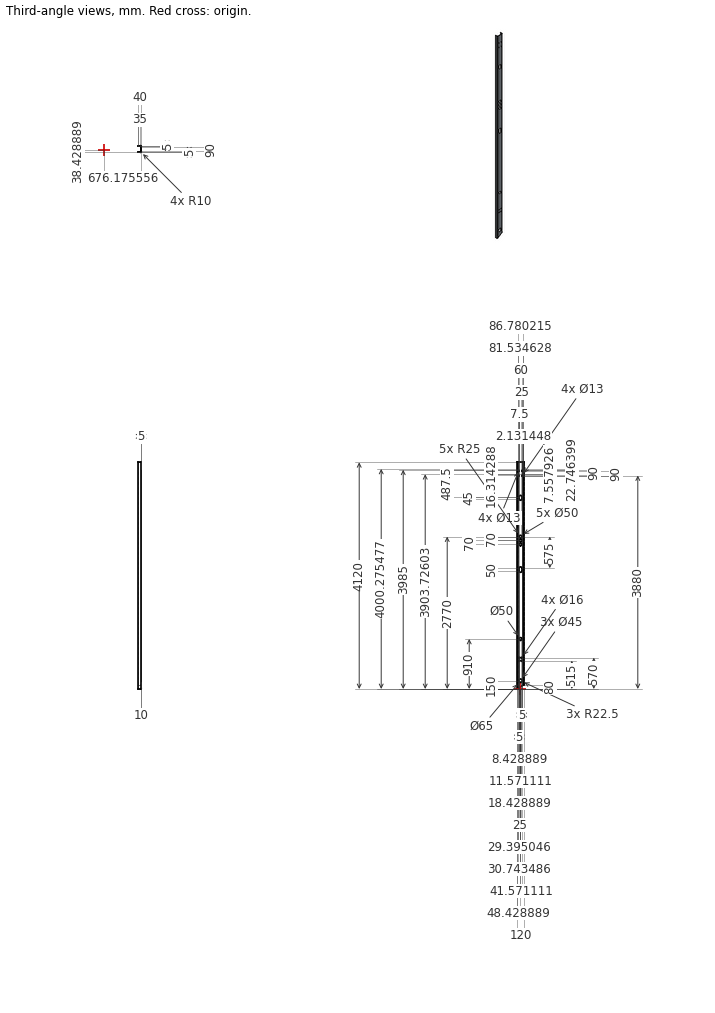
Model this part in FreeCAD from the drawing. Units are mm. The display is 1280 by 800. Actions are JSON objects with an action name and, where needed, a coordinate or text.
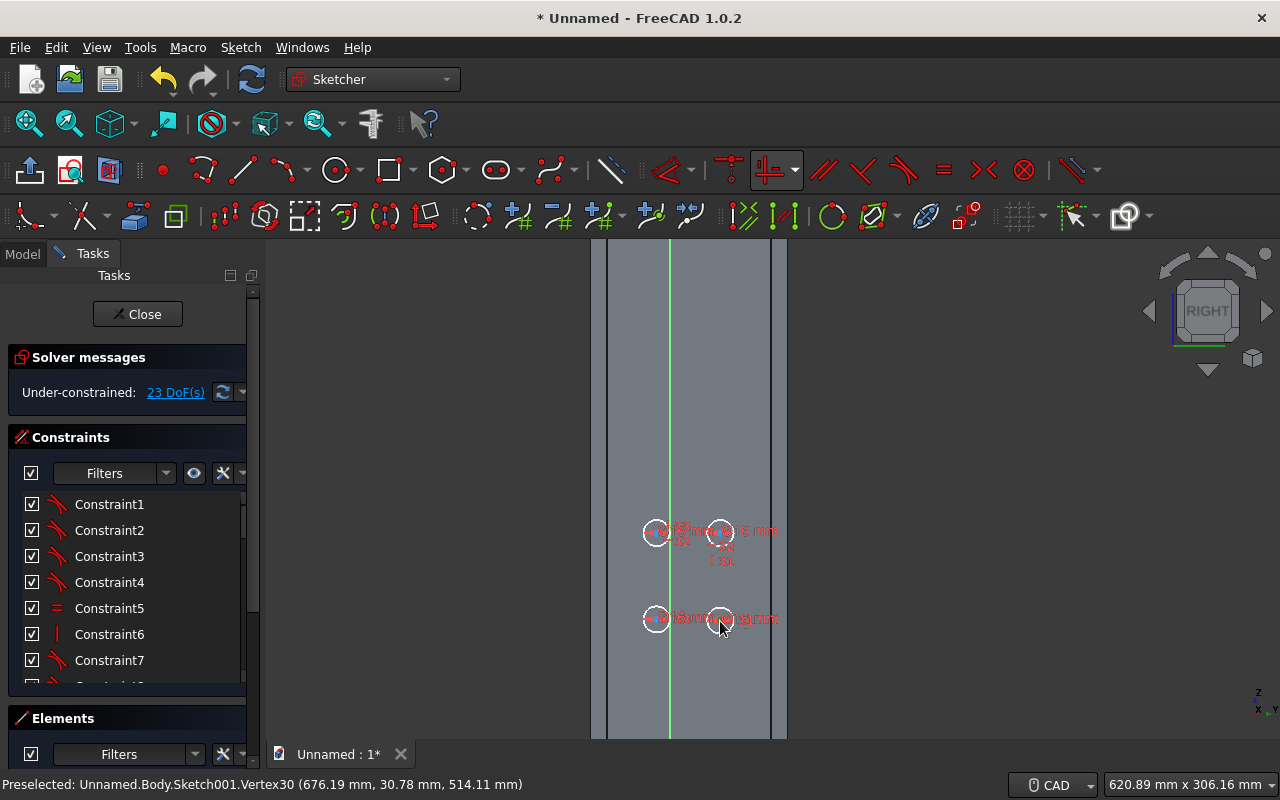
{"action": "scroll", "coordinate": [705, 609], "scroll_direction": "down", "scroll_amount": 15}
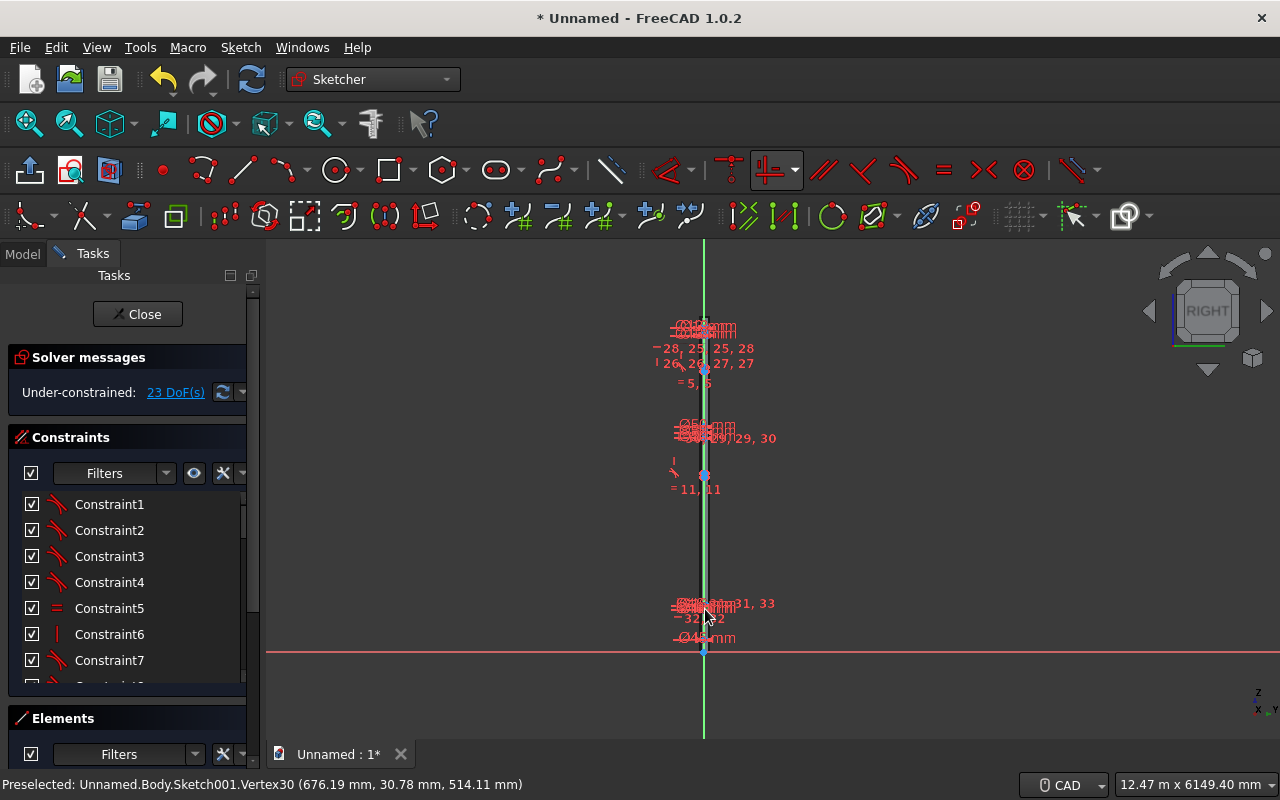
{"action": "scroll", "coordinate": [703, 610], "scroll_direction": "up", "scroll_amount": 7}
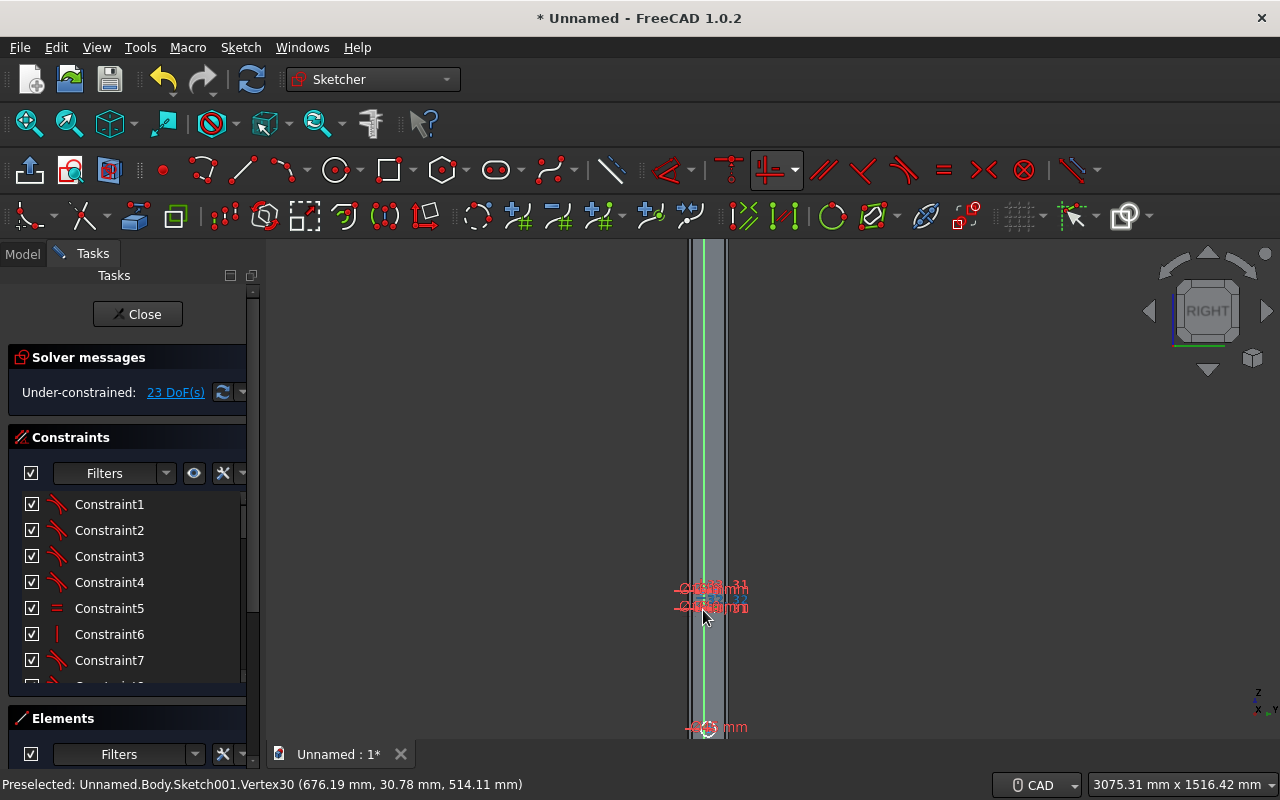
{"action": "scroll", "coordinate": [702, 609], "scroll_direction": "up", "scroll_amount": 4}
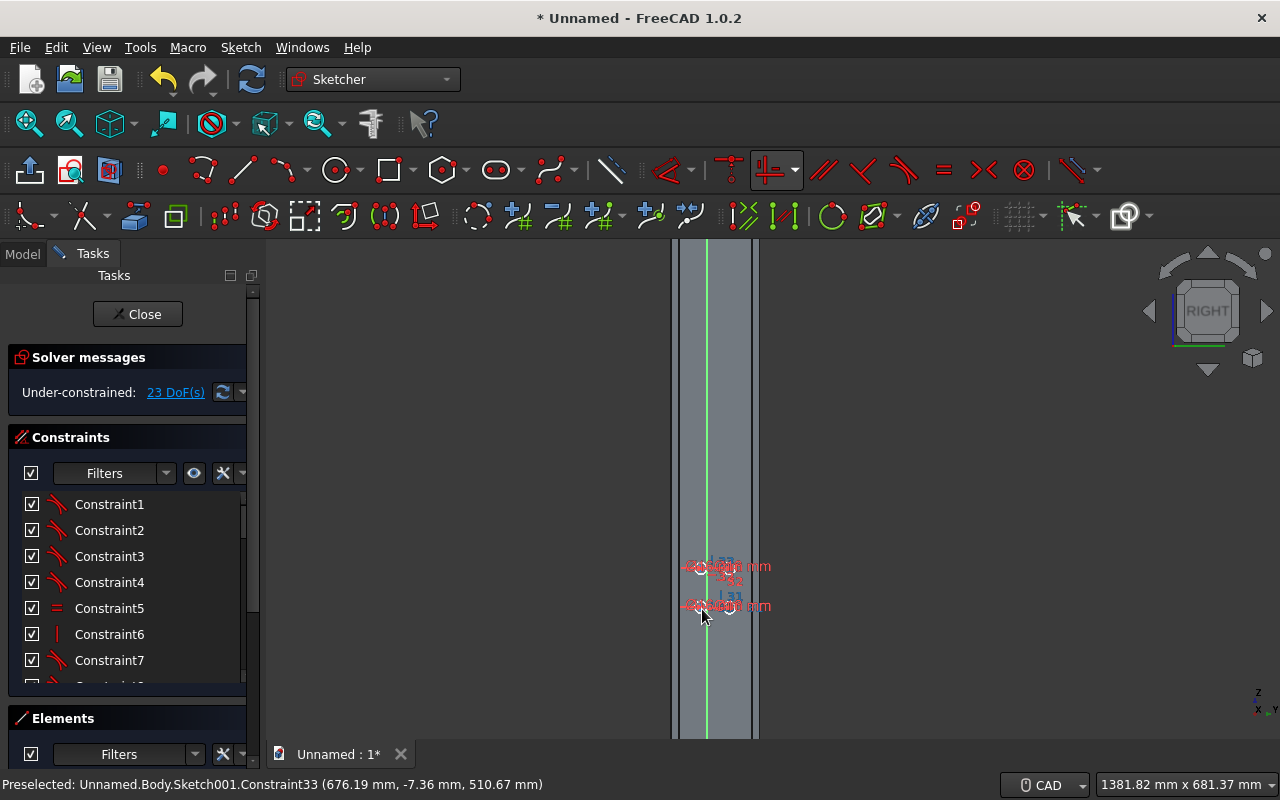
{"action": "left_click", "coordinate": [701, 607]}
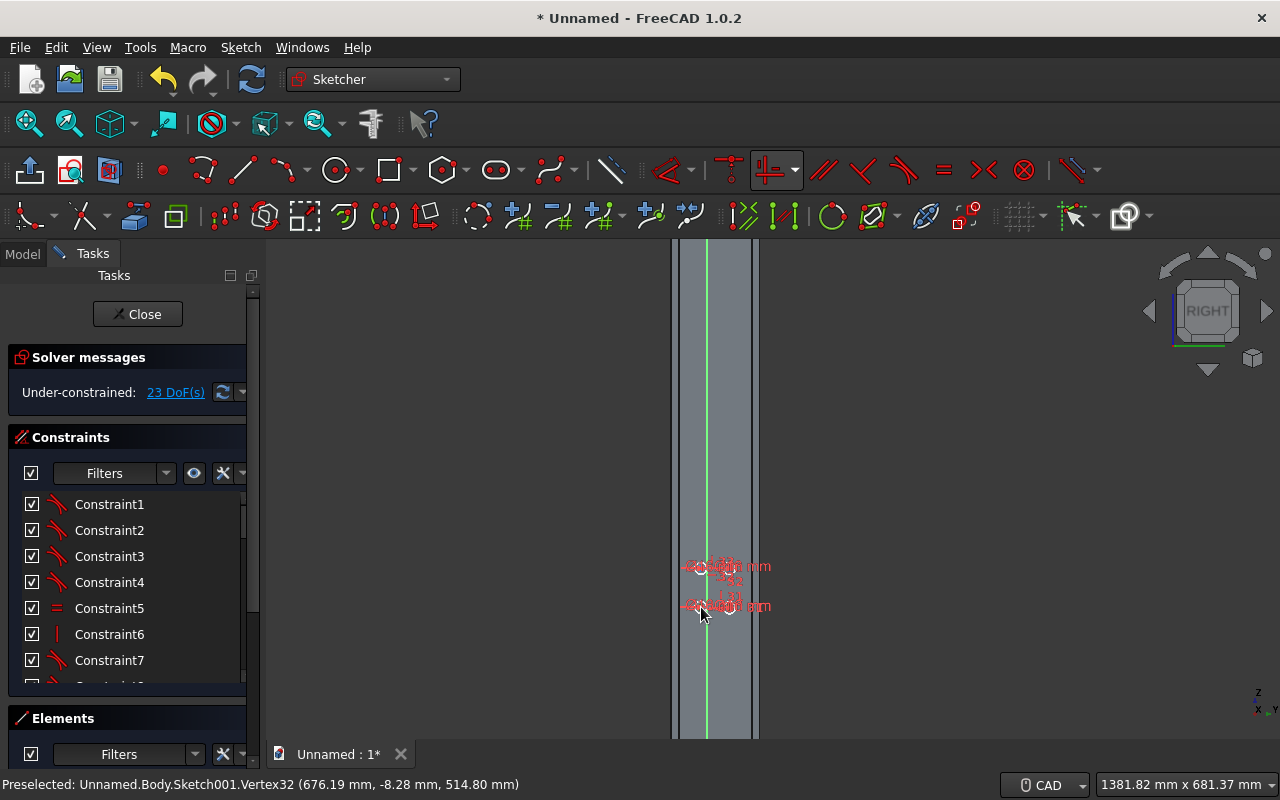
{"action": "key", "text": "h"}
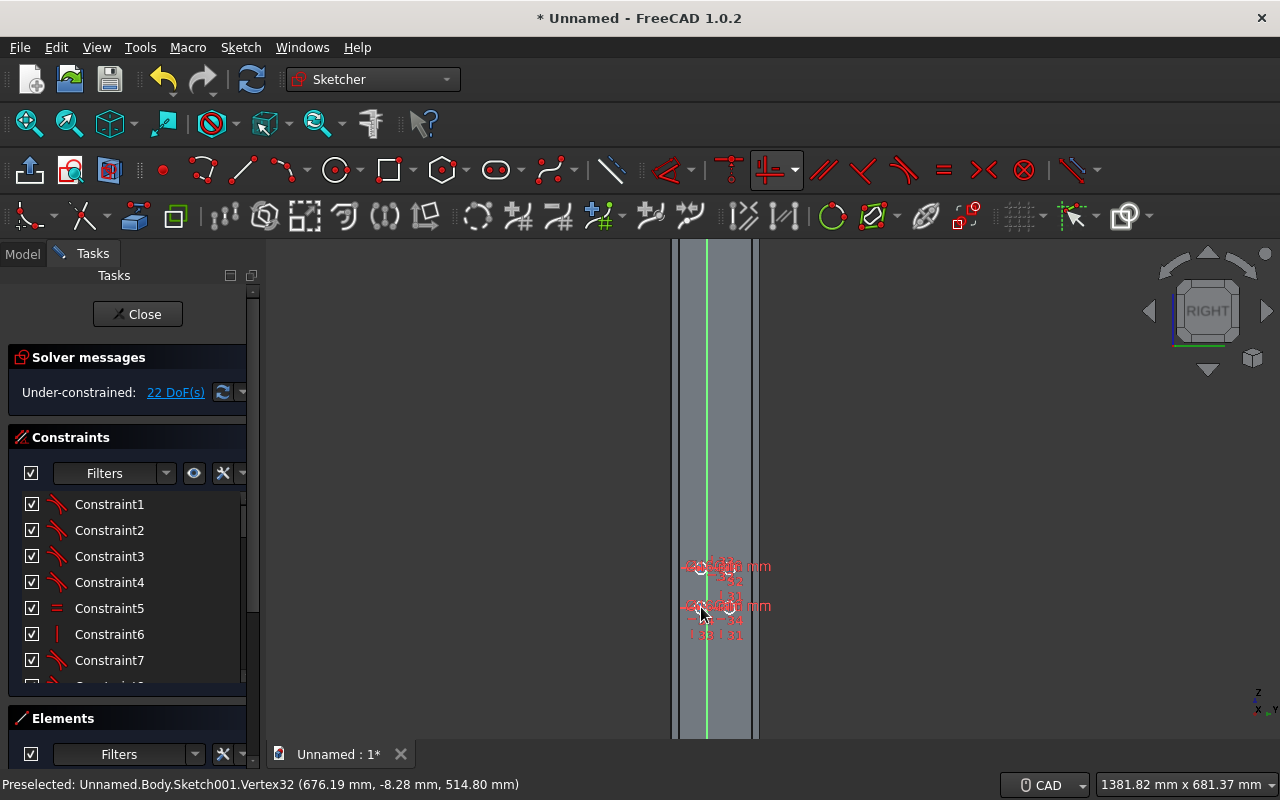
{"action": "key", "text": "d"}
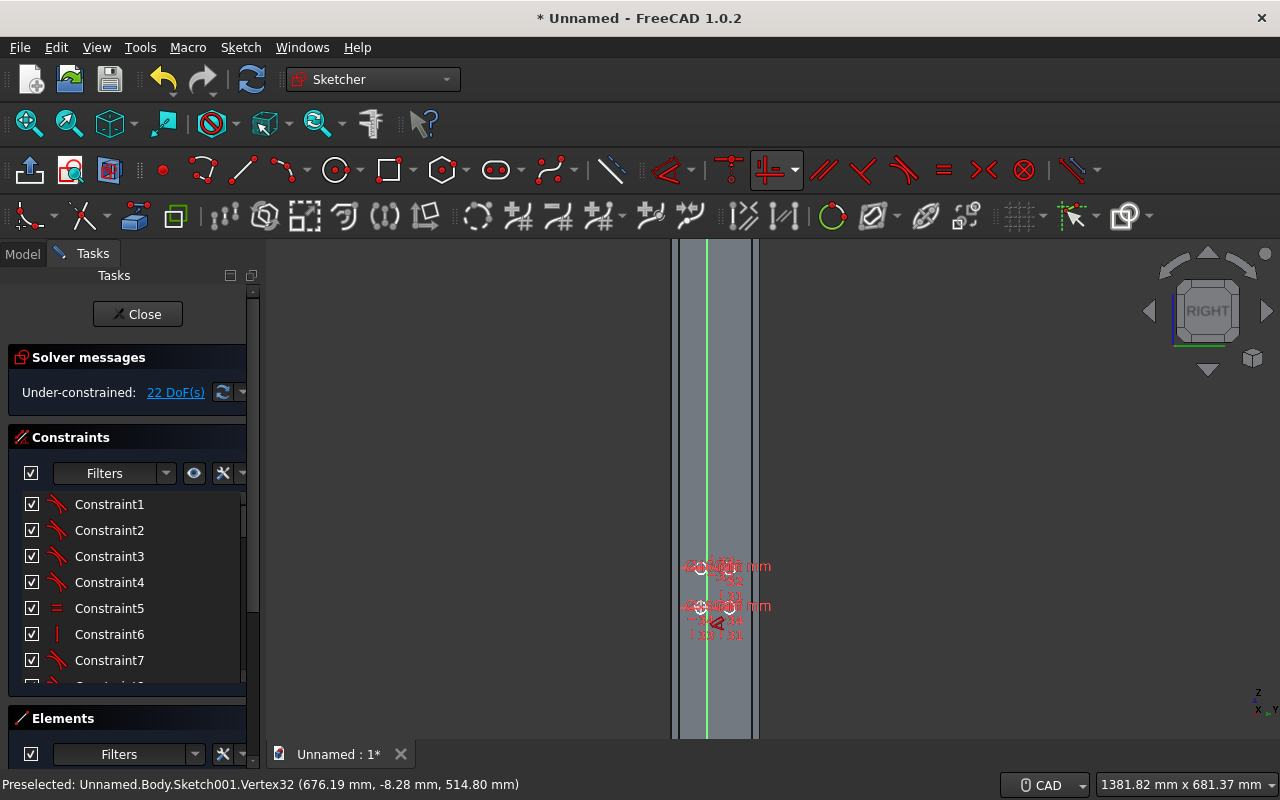
{"action": "scroll", "coordinate": [703, 610], "scroll_direction": "down", "scroll_amount": 11}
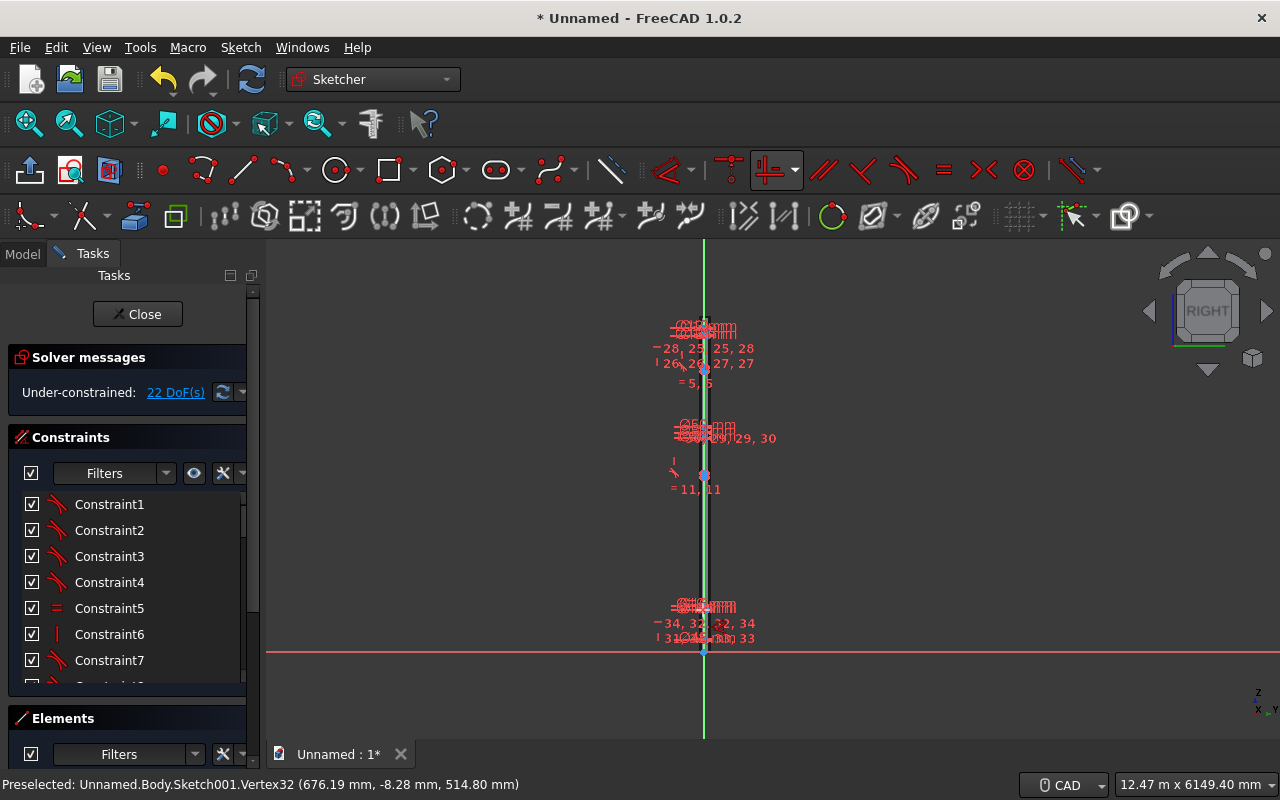
{"action": "scroll", "coordinate": [704, 373], "scroll_direction": "up", "scroll_amount": 16}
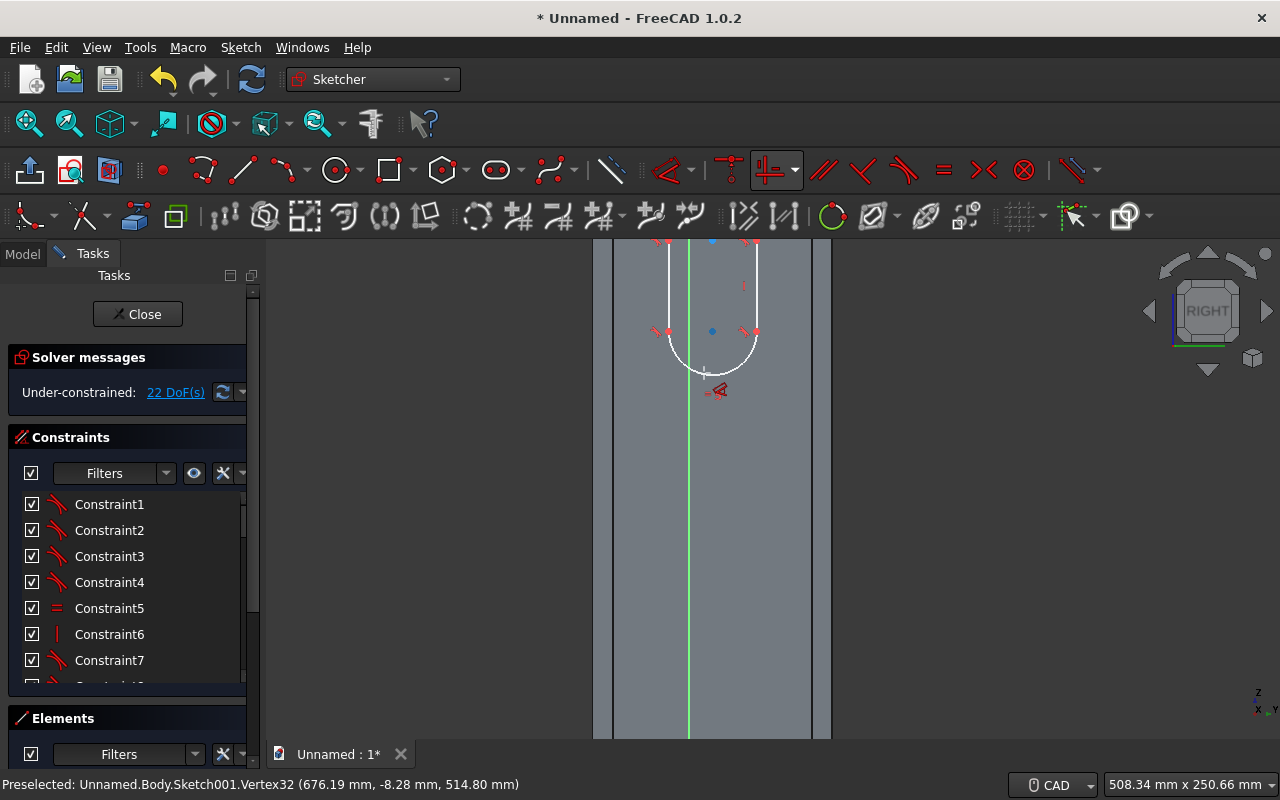
{"action": "left_click", "coordinate": [687, 367]}
{"action": "left_click", "coordinate": [668, 393]}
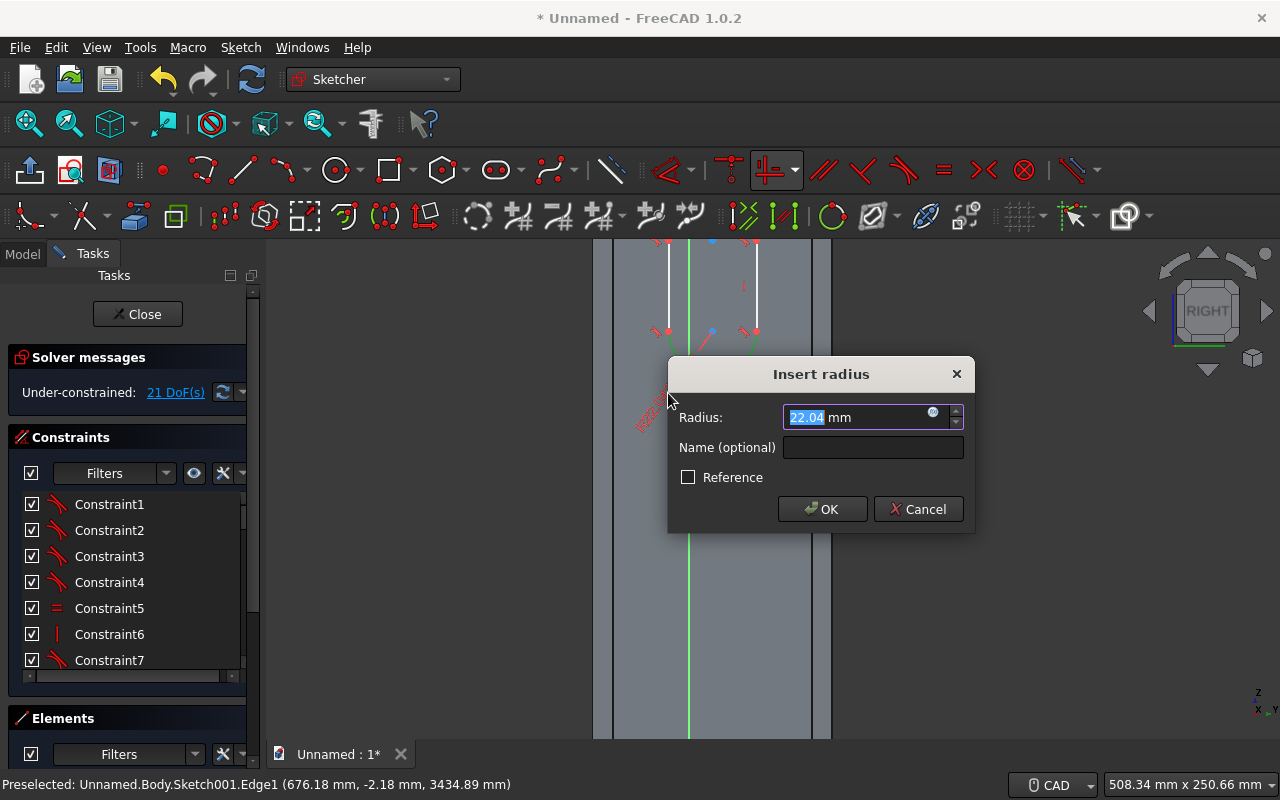
{"action": "type", "text": "22.5"}
{"action": "key", "text": "Return"}